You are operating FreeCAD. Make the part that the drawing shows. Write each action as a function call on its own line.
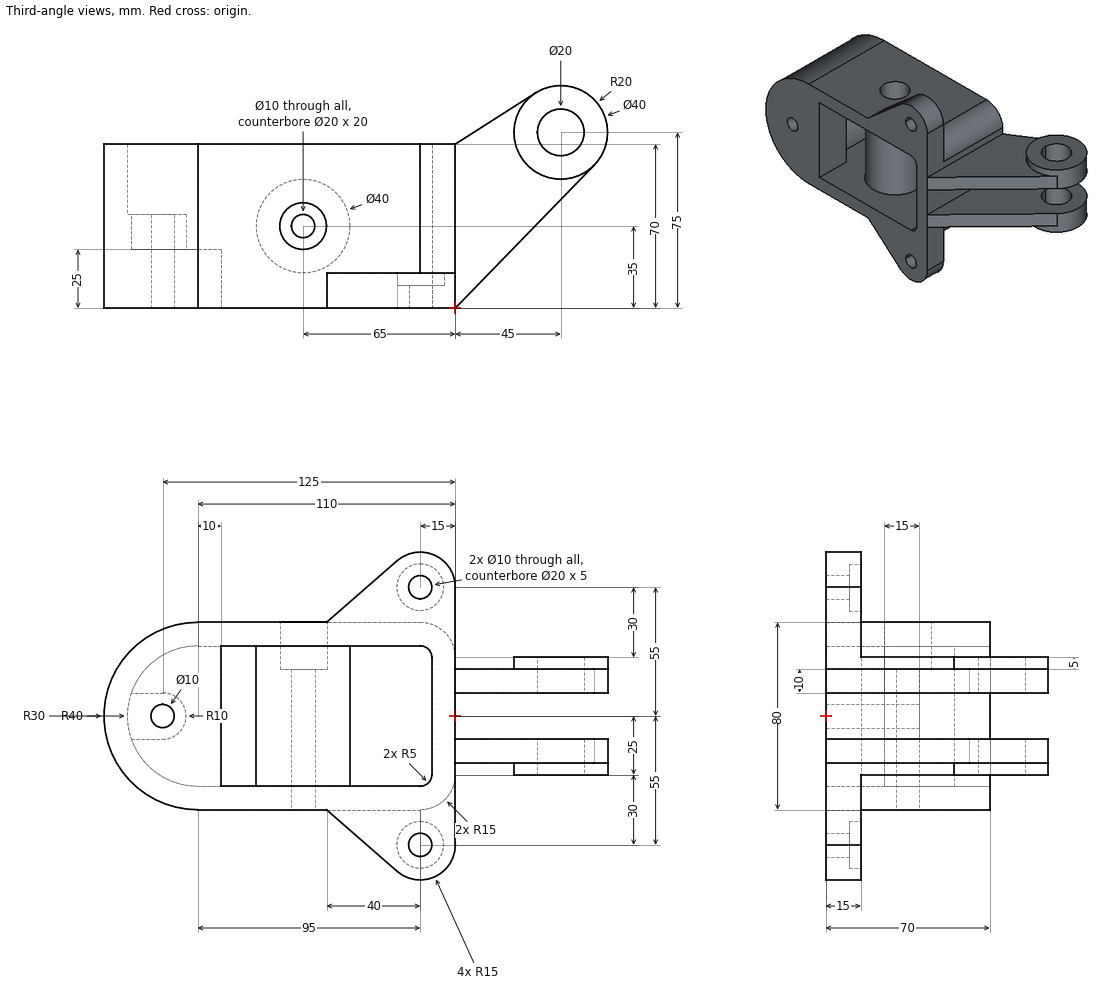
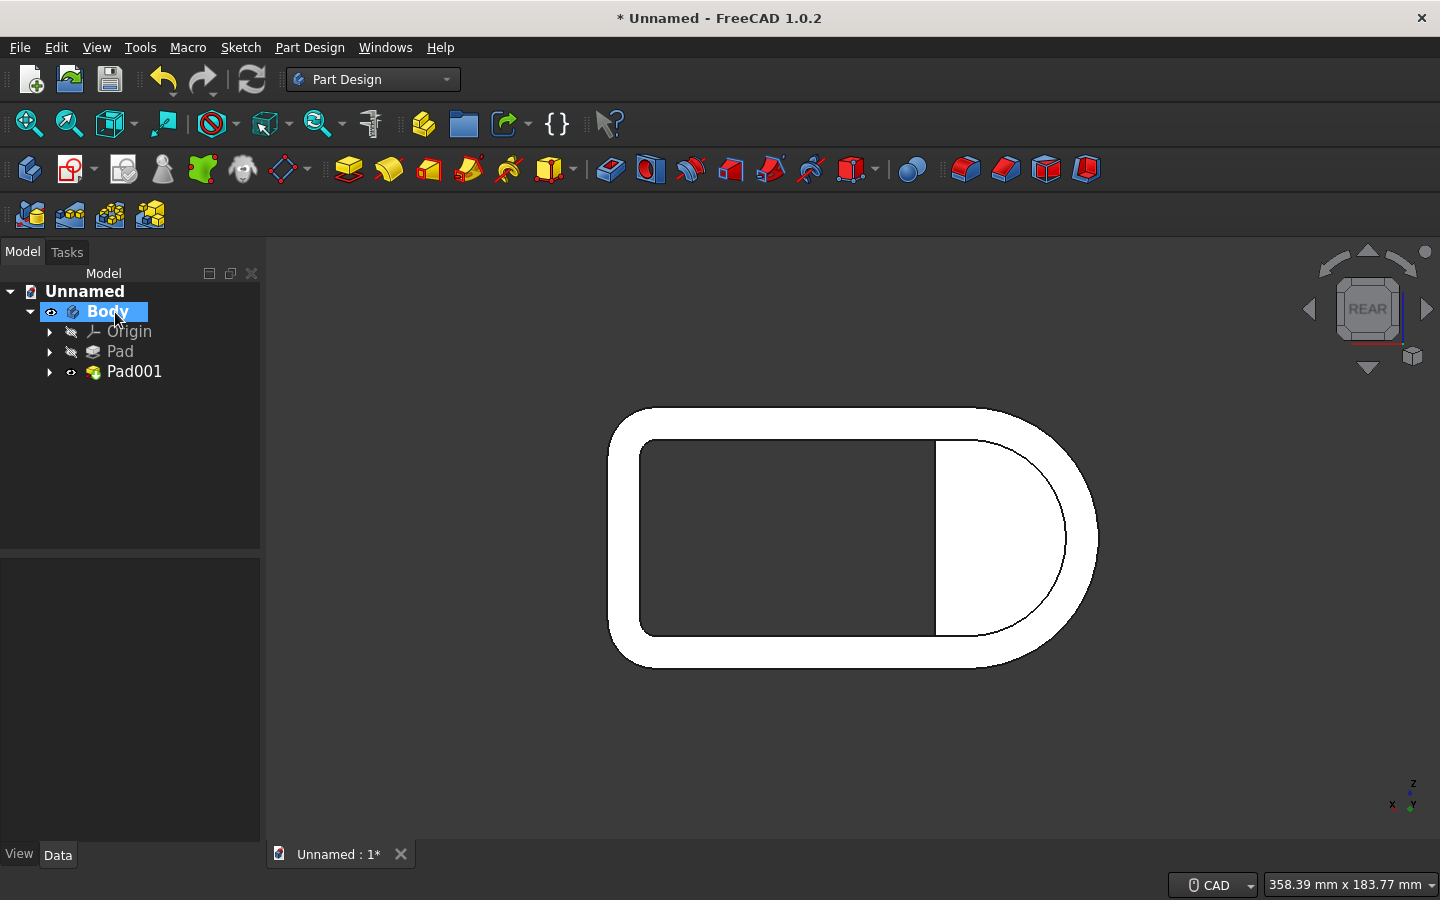
click(30, 124)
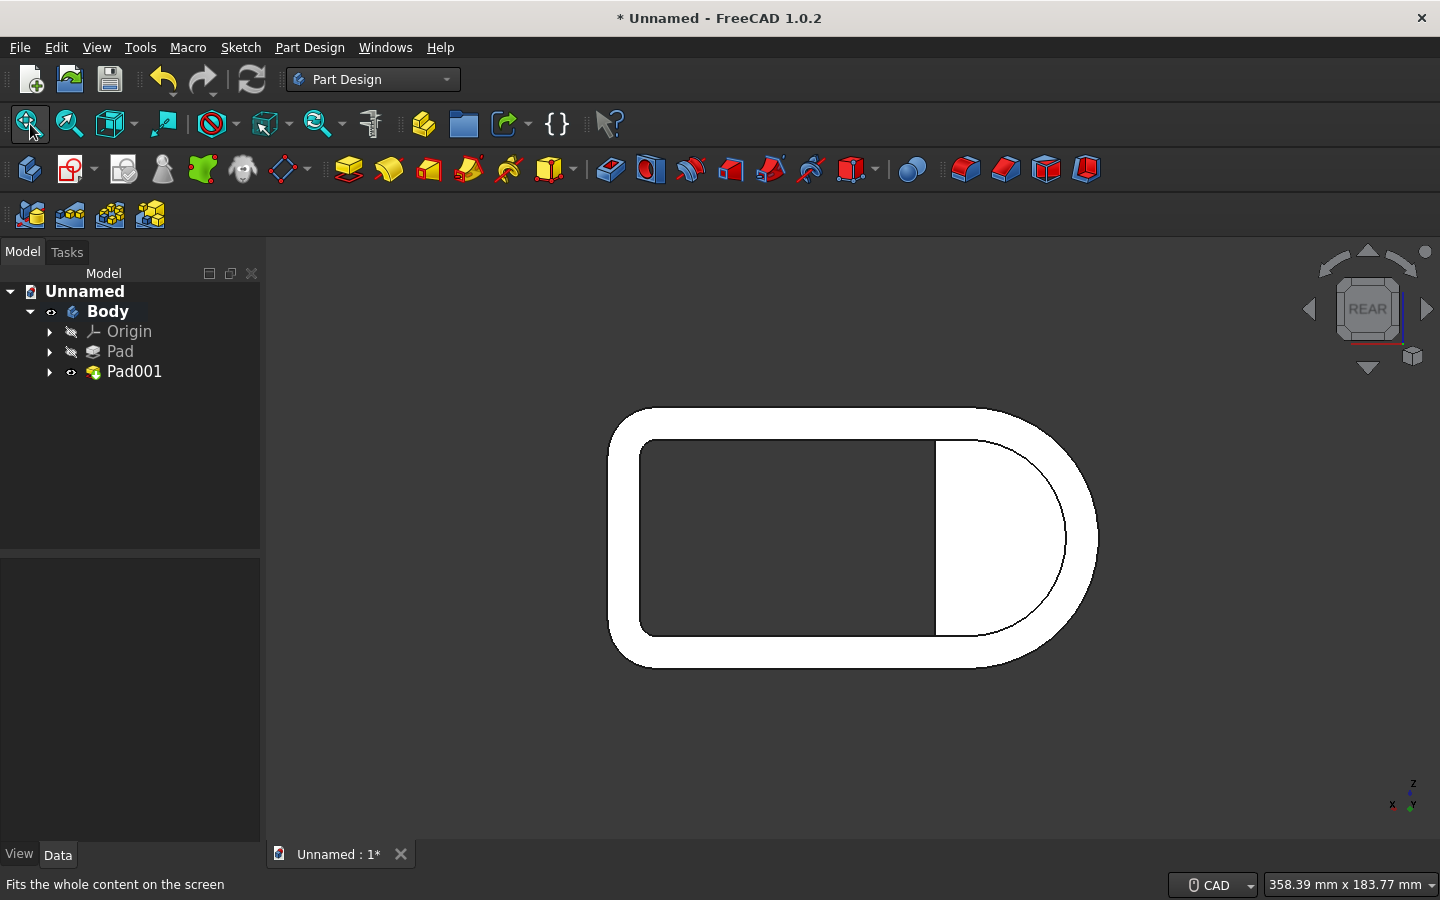
click(1001, 537)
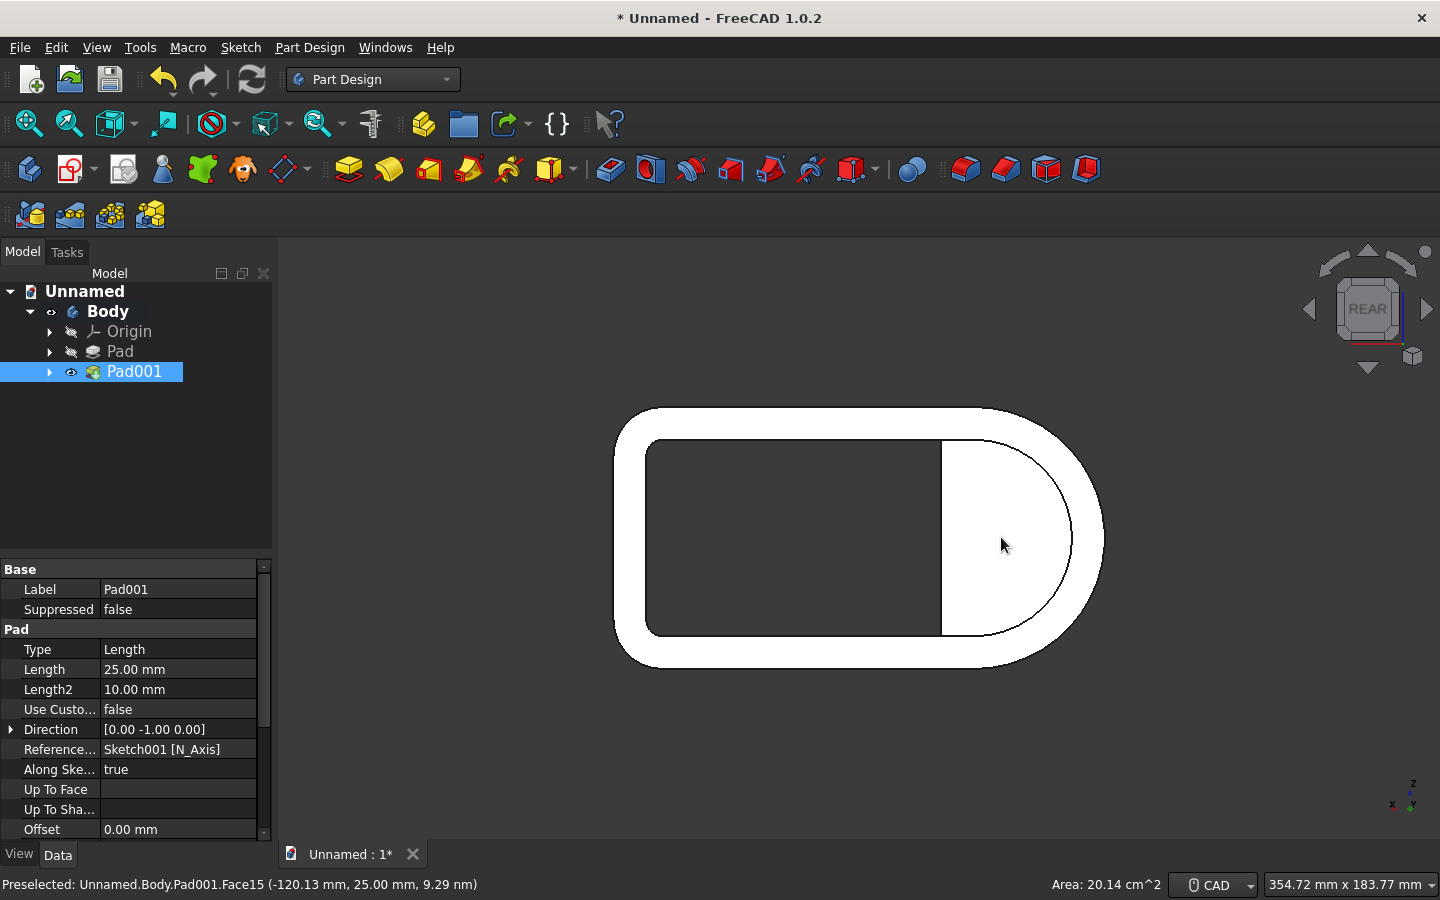
click(70, 170)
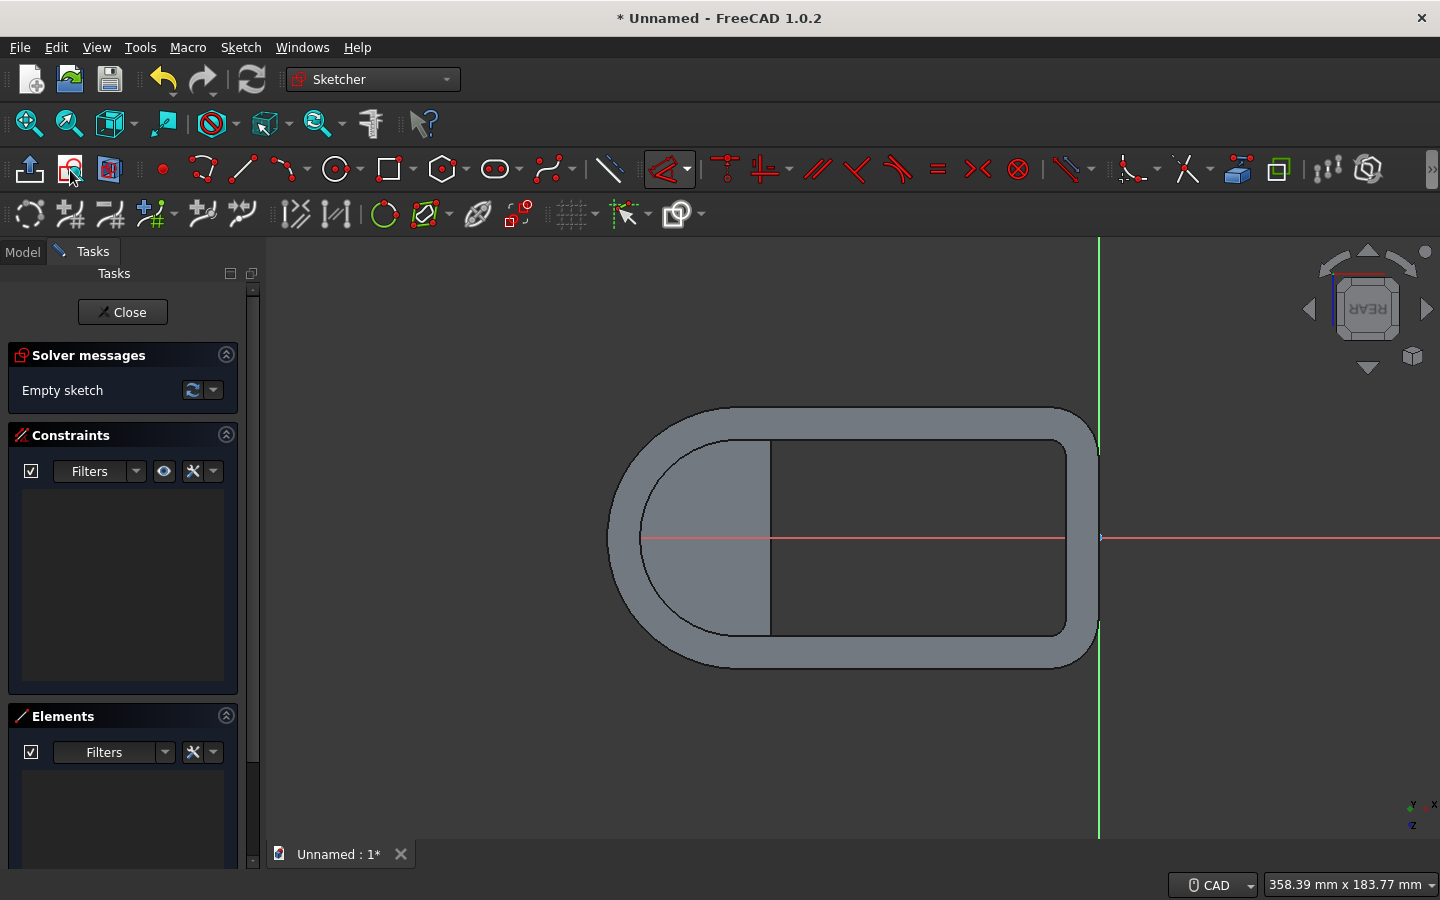
click(110, 170)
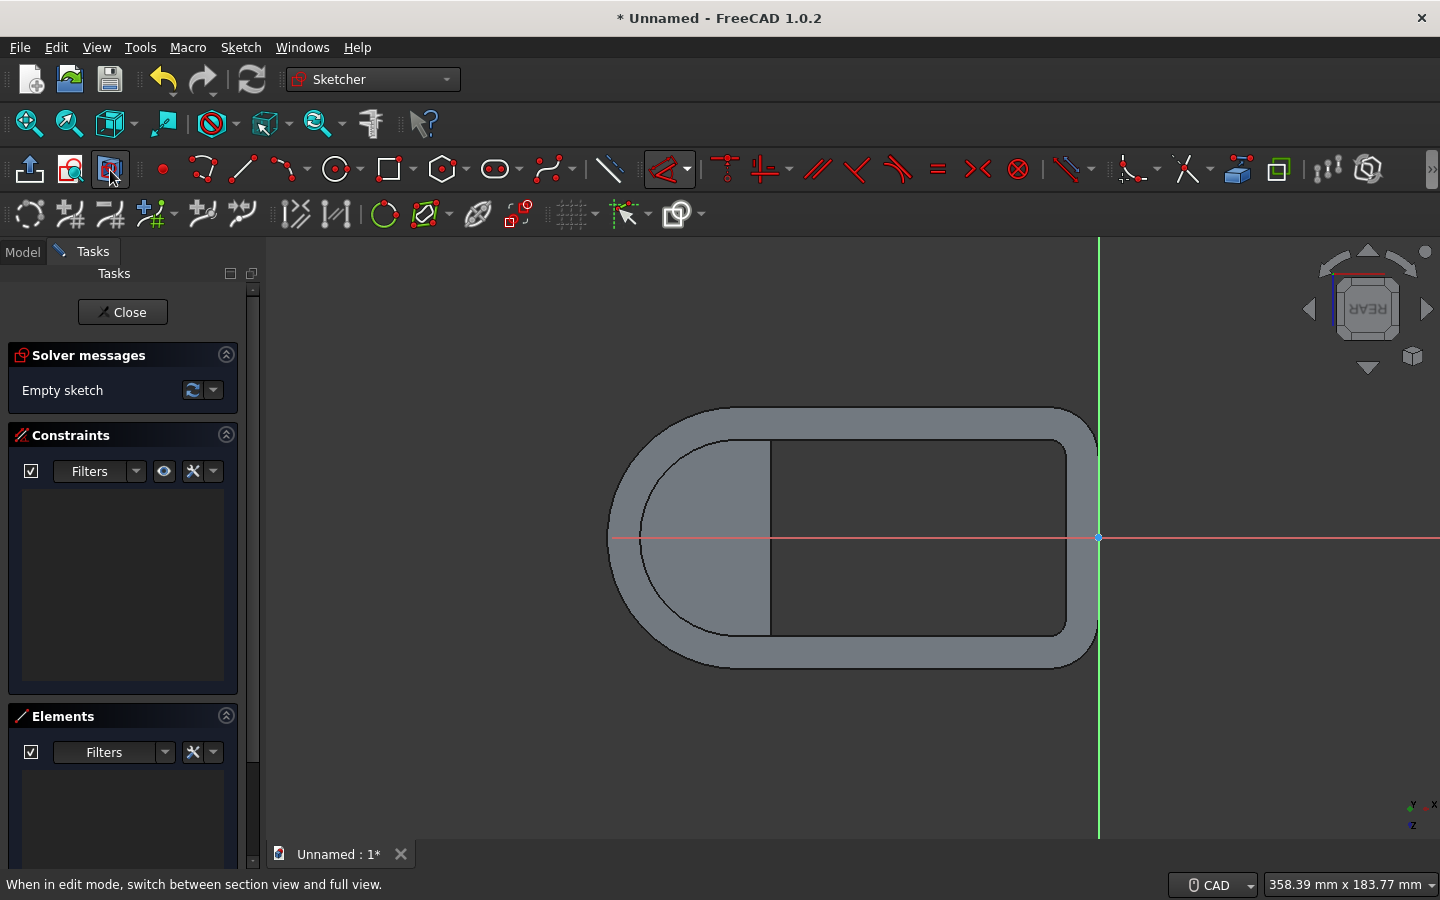
scroll(660, 538, up, 9)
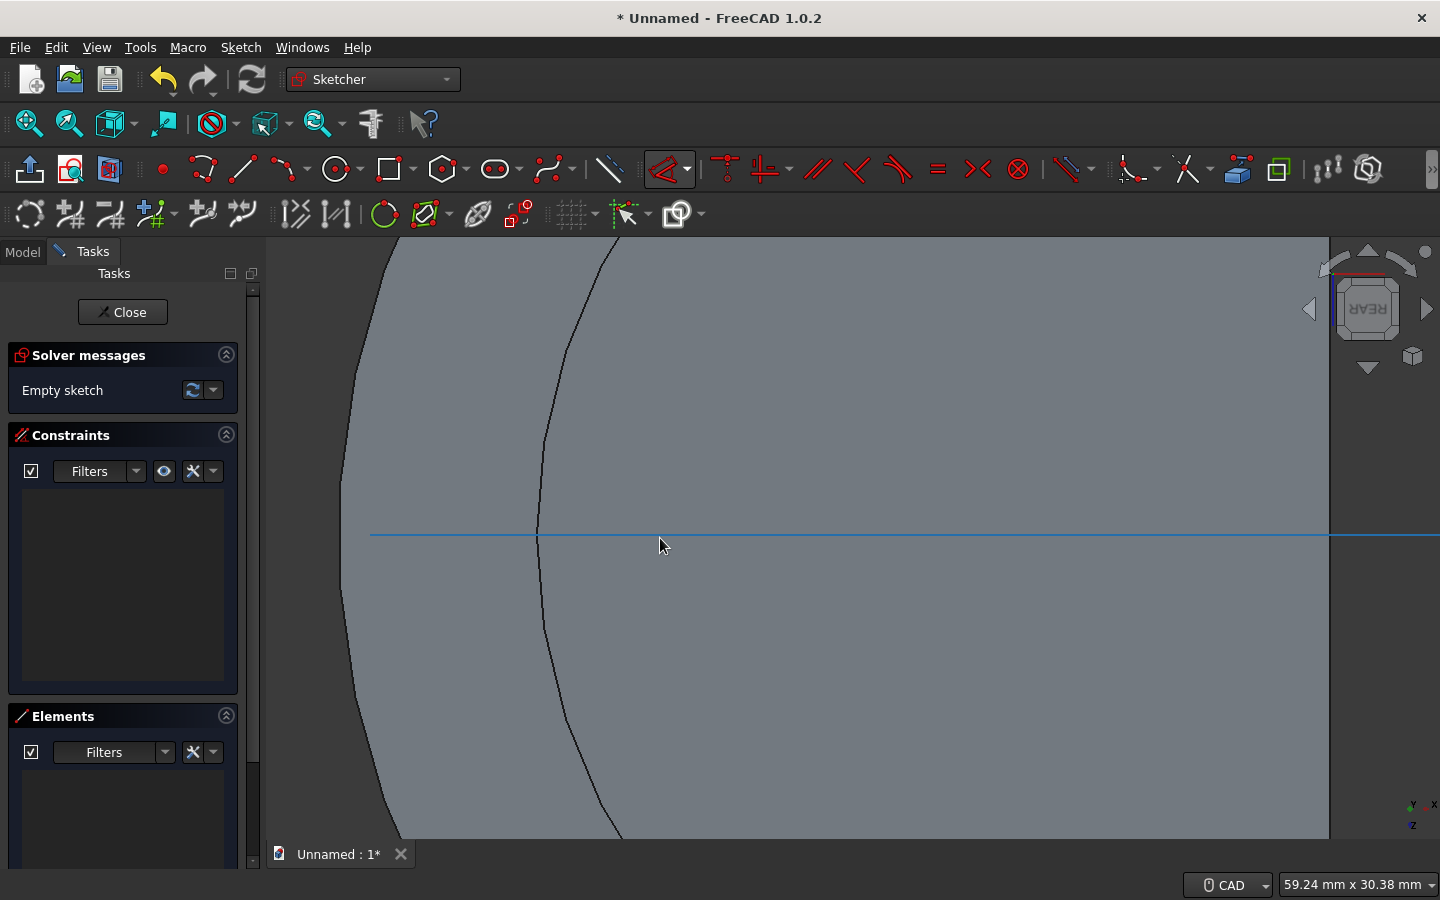
key(g)
key(l)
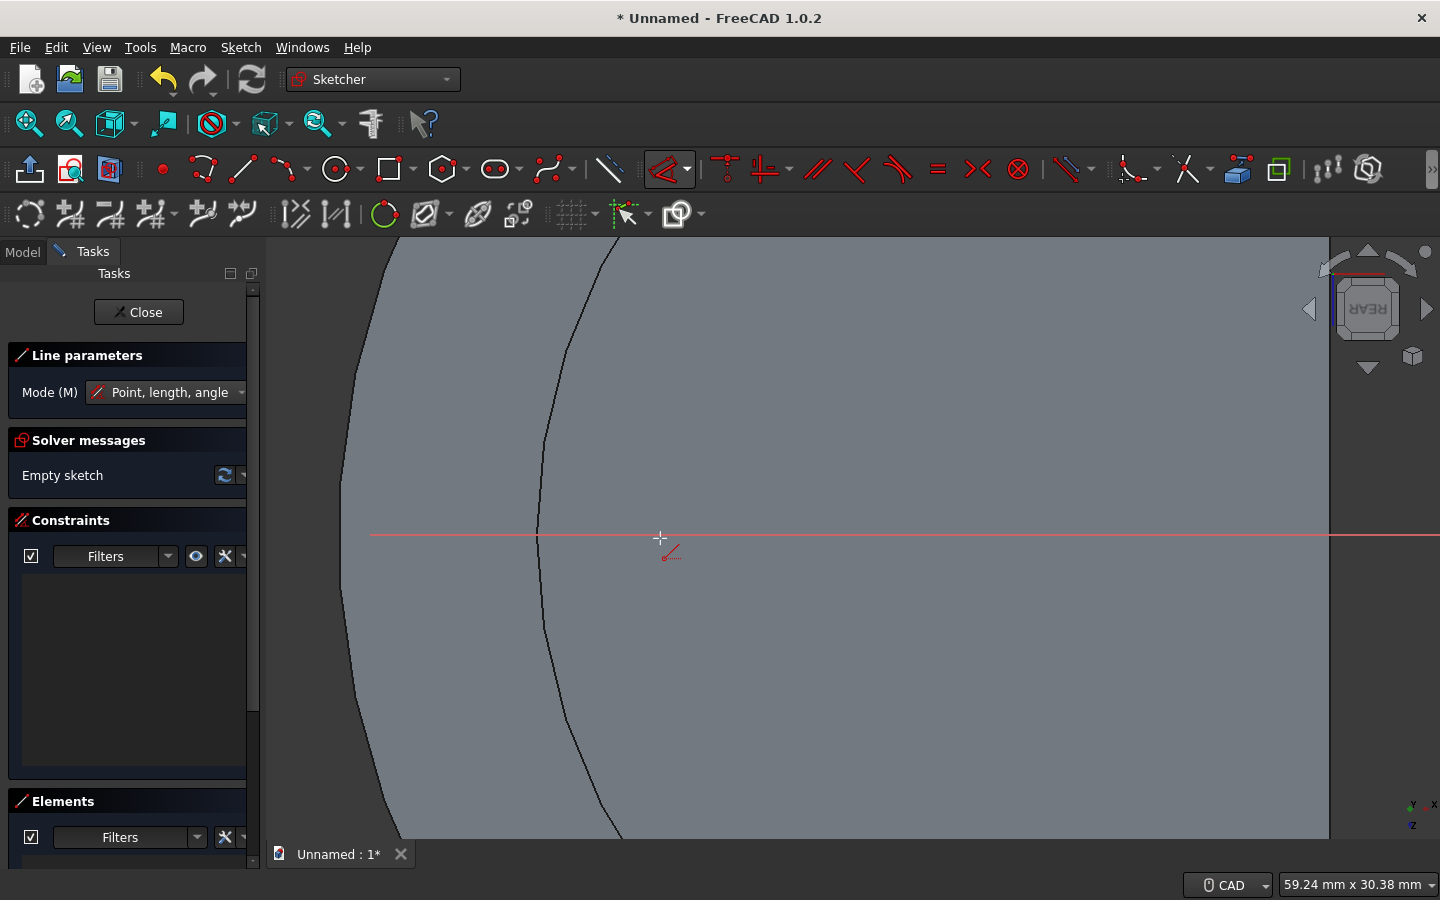
click(571, 734)
click(834, 734)